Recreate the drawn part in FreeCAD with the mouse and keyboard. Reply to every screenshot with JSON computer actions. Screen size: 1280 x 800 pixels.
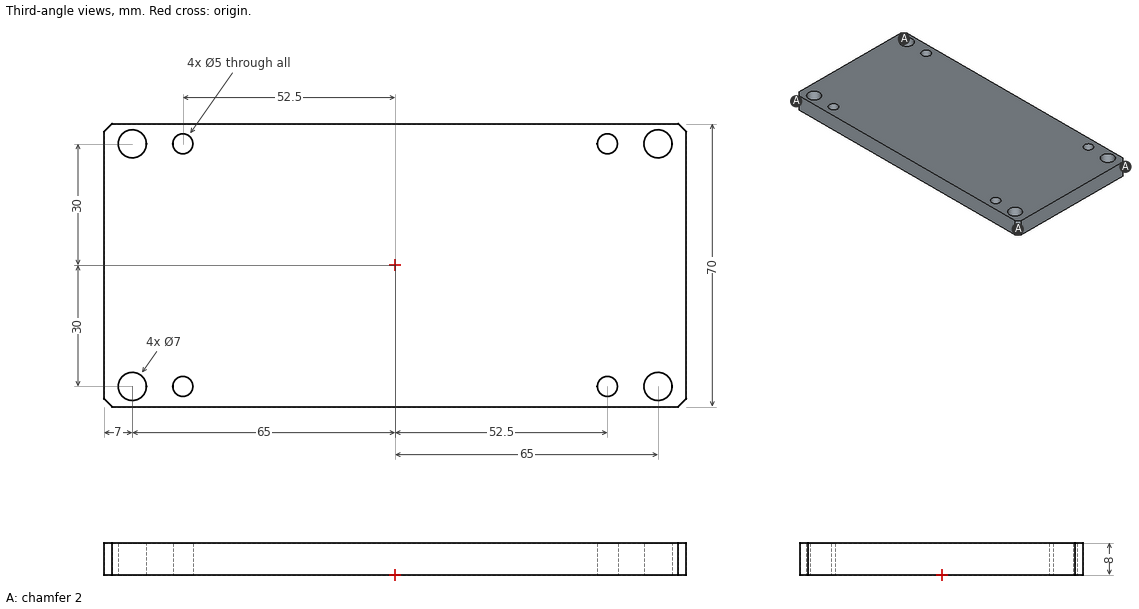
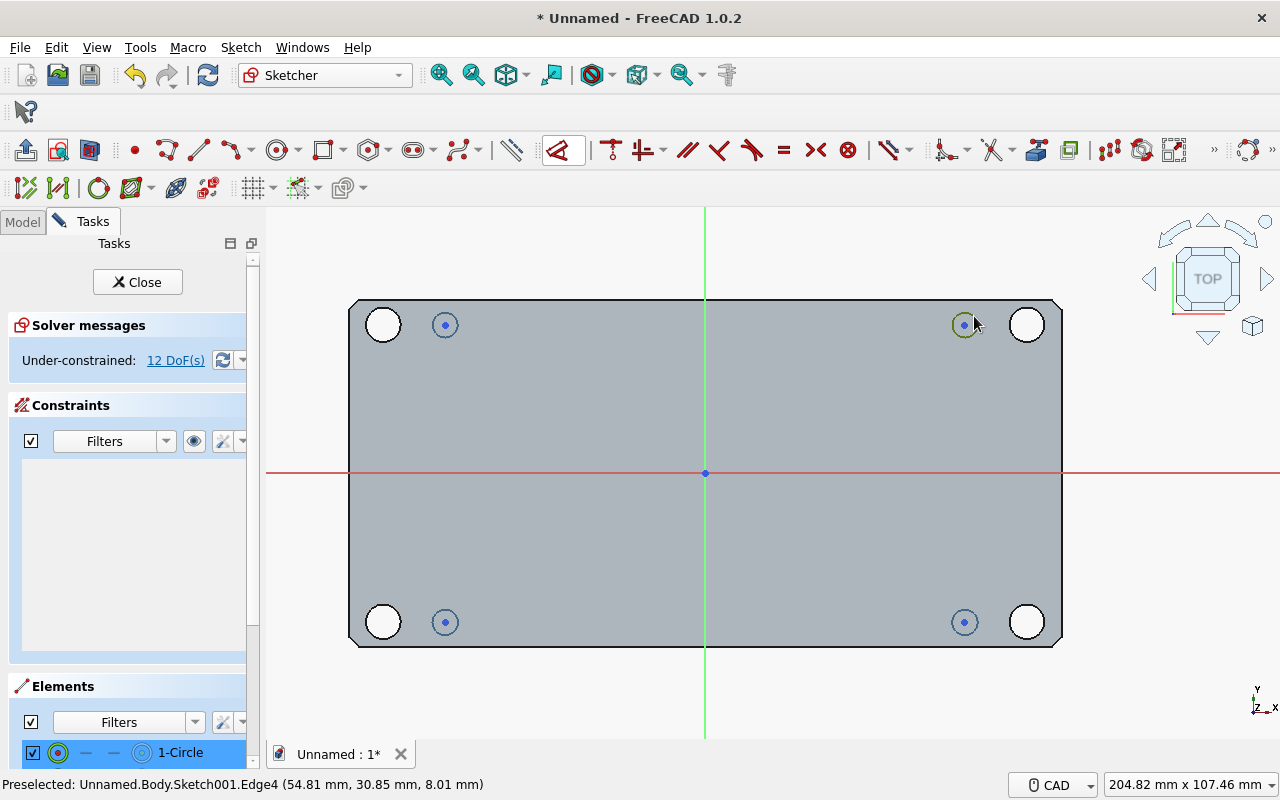
{"action": "left_click", "coordinate": [784, 150]}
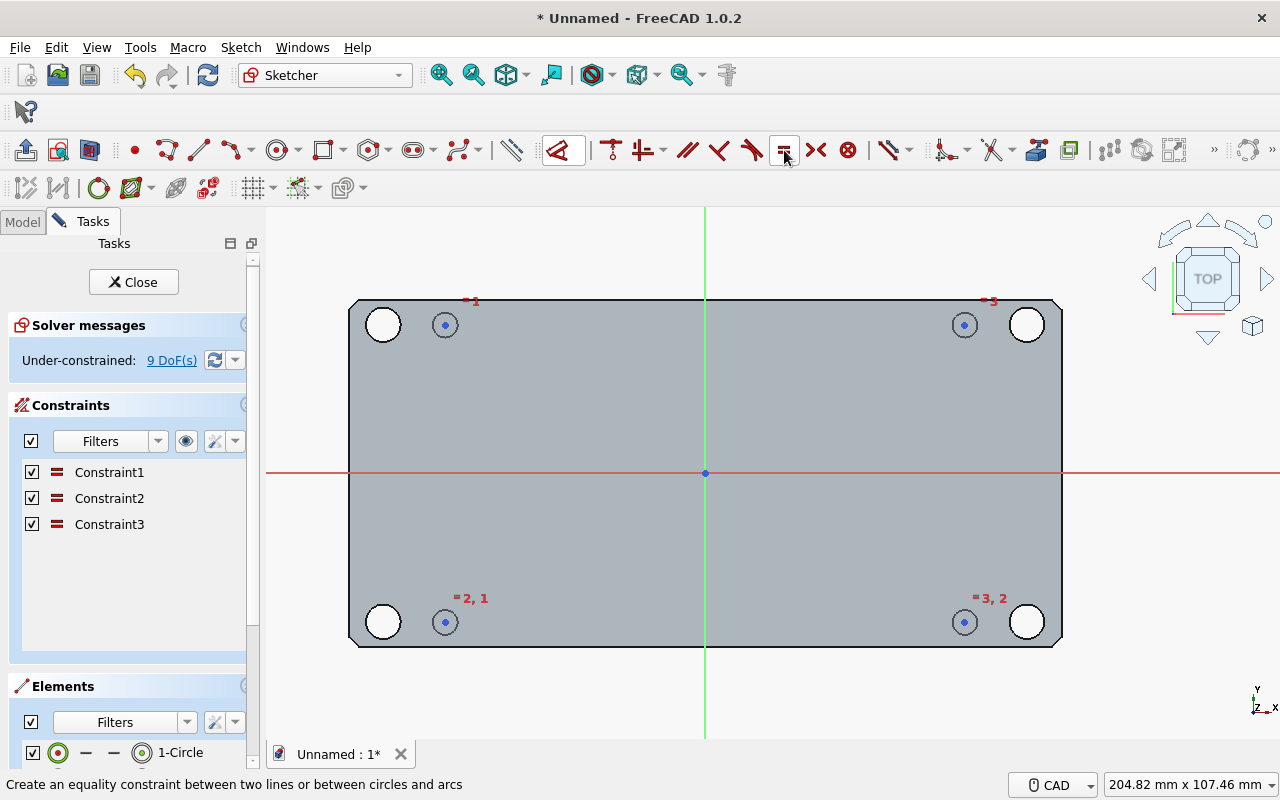
{"action": "scroll", "coordinate": [454, 316], "scroll_direction": "up", "scroll_amount": 3}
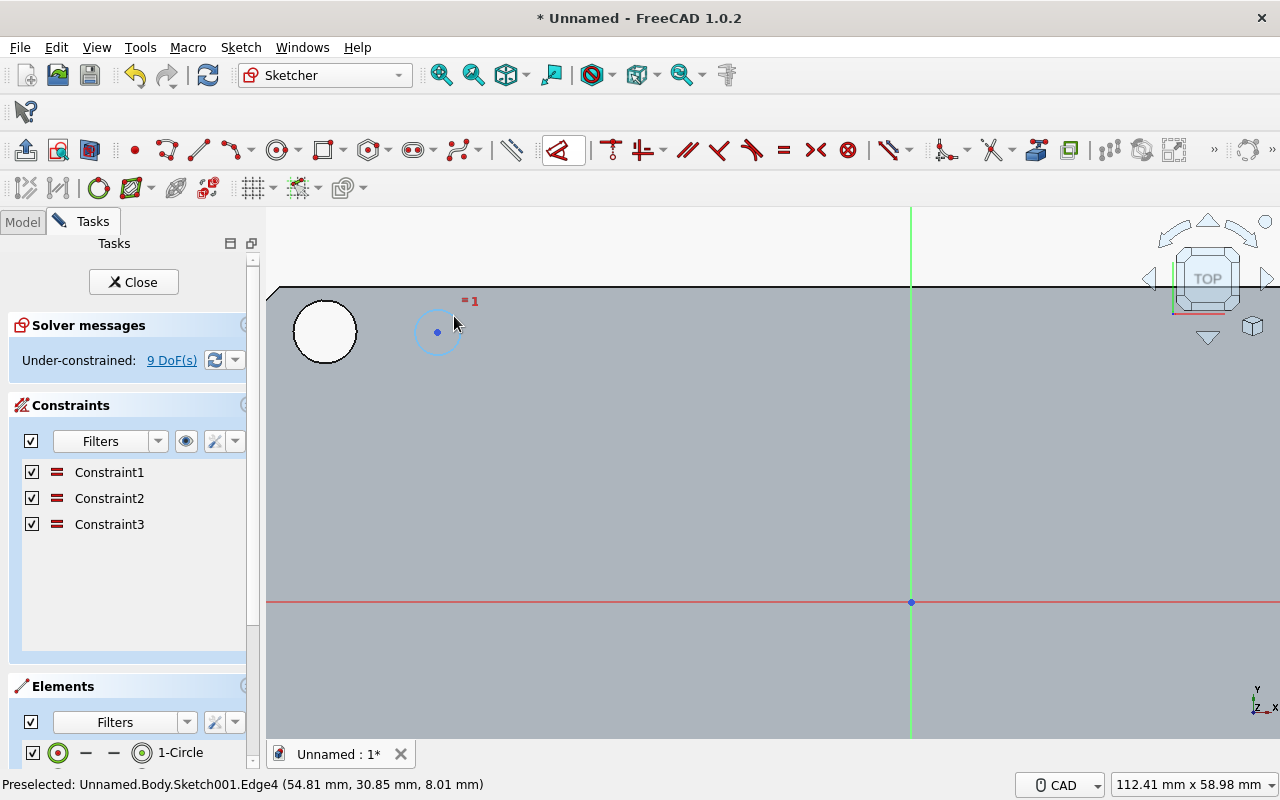
{"action": "left_click", "coordinate": [454, 316]}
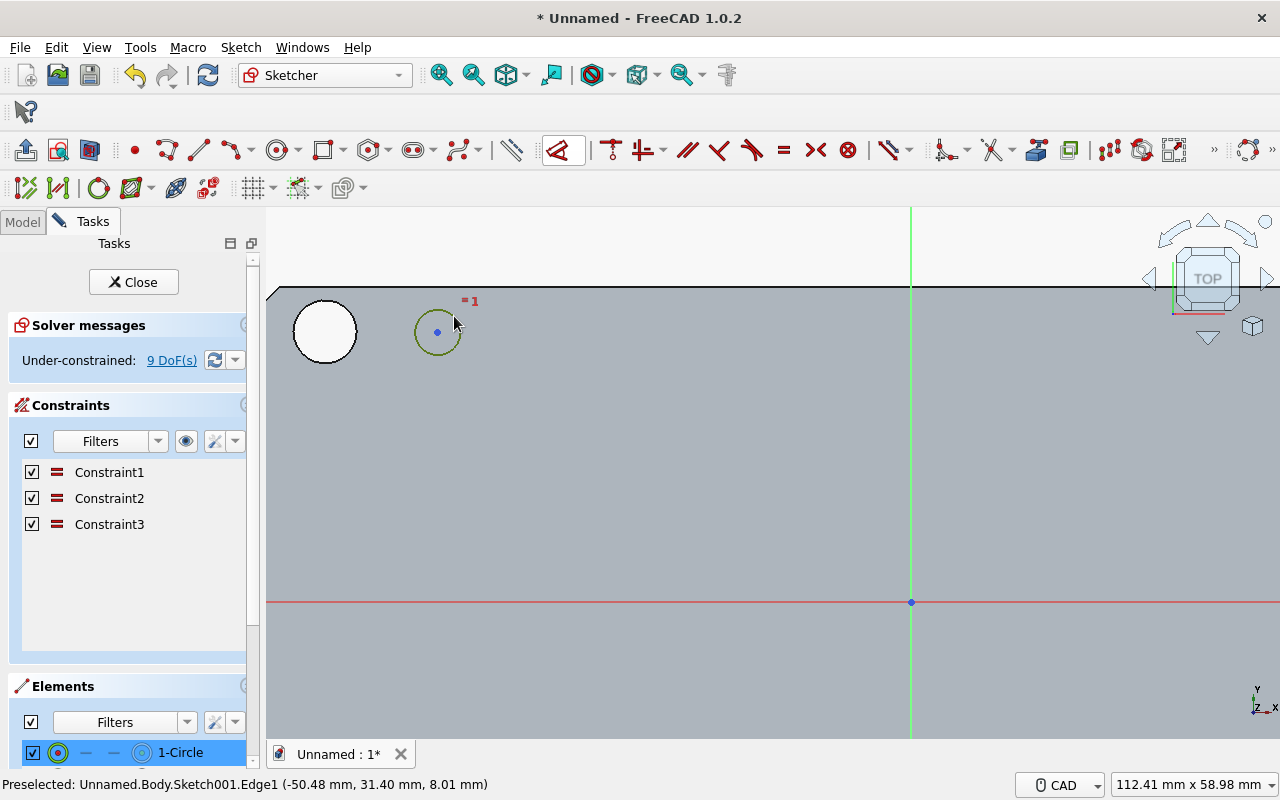
{"action": "key", "text": "k o"}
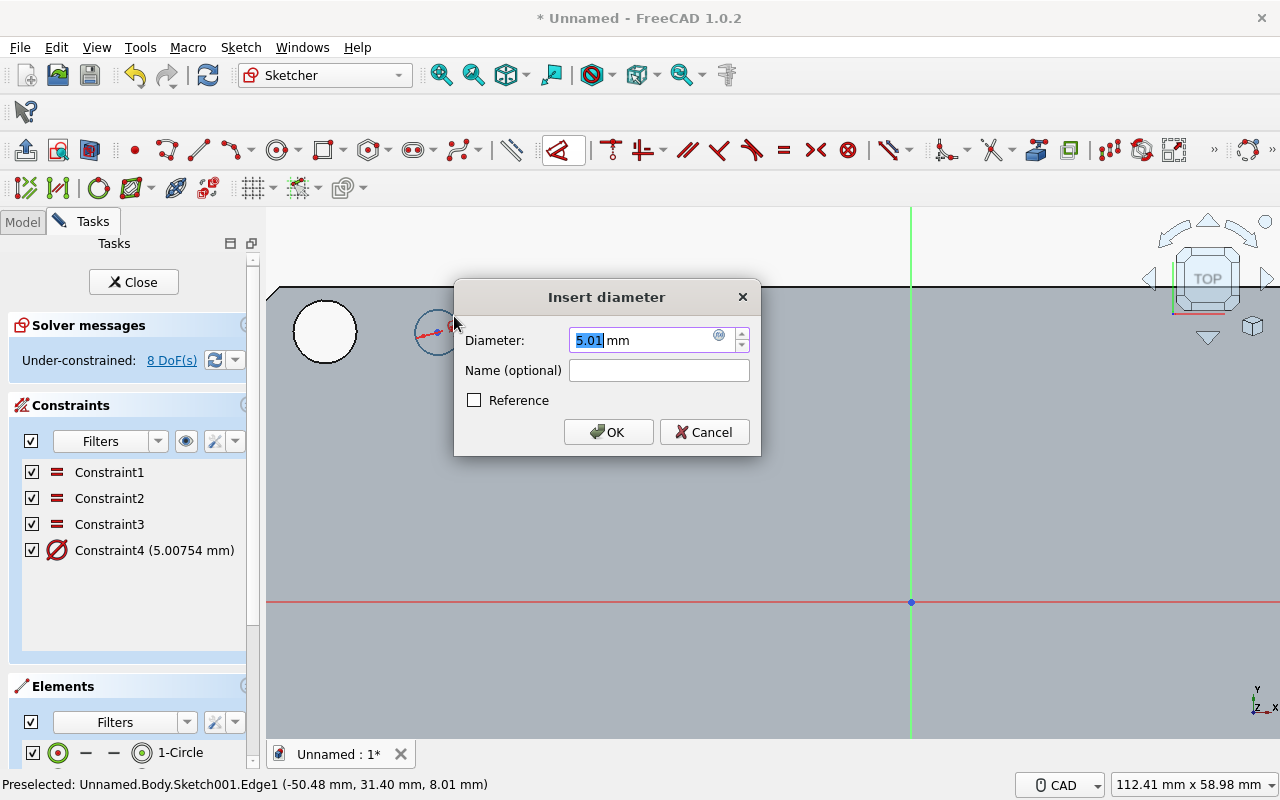
{"action": "type", "text": "5"}
{"action": "key", "text": "Return"}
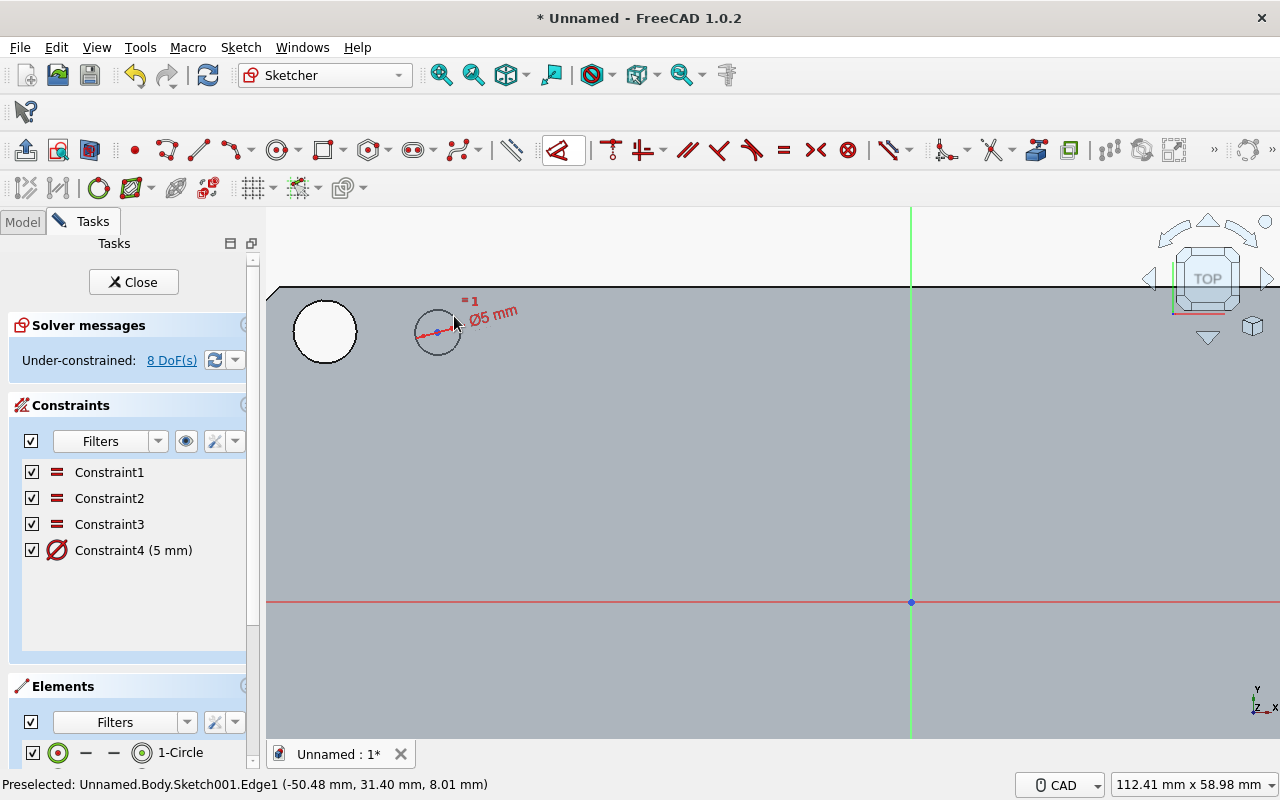
{"action": "left_click", "coordinate": [438, 332]}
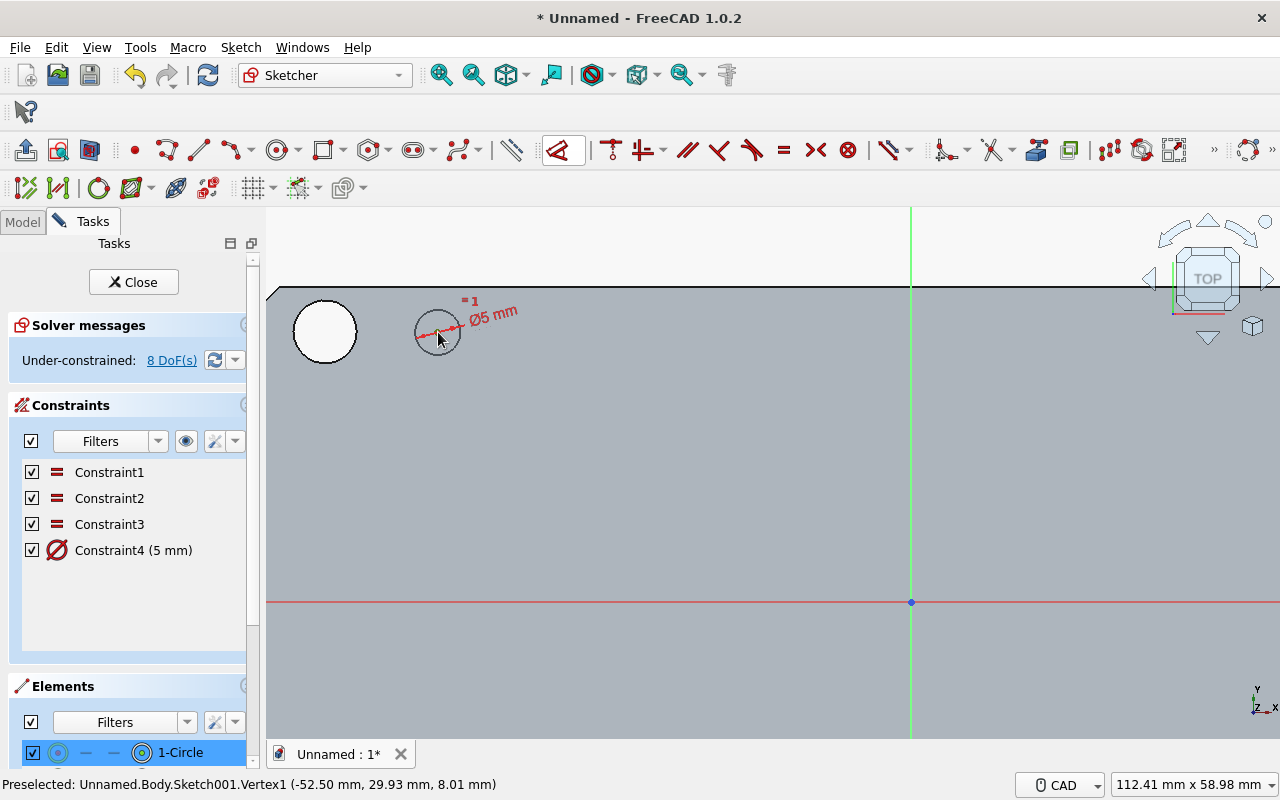
{"action": "left_click", "coordinate": [580, 150]}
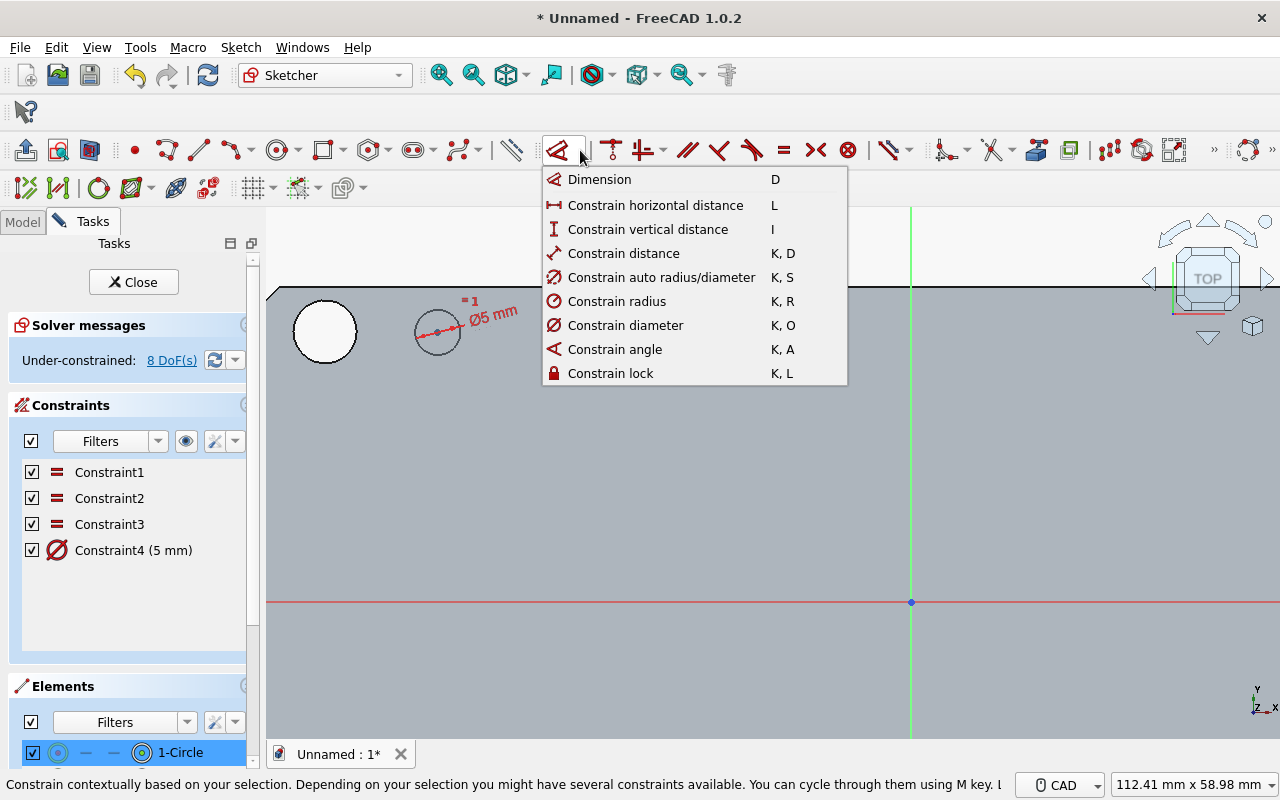
{"action": "left_click", "coordinate": [695, 229]}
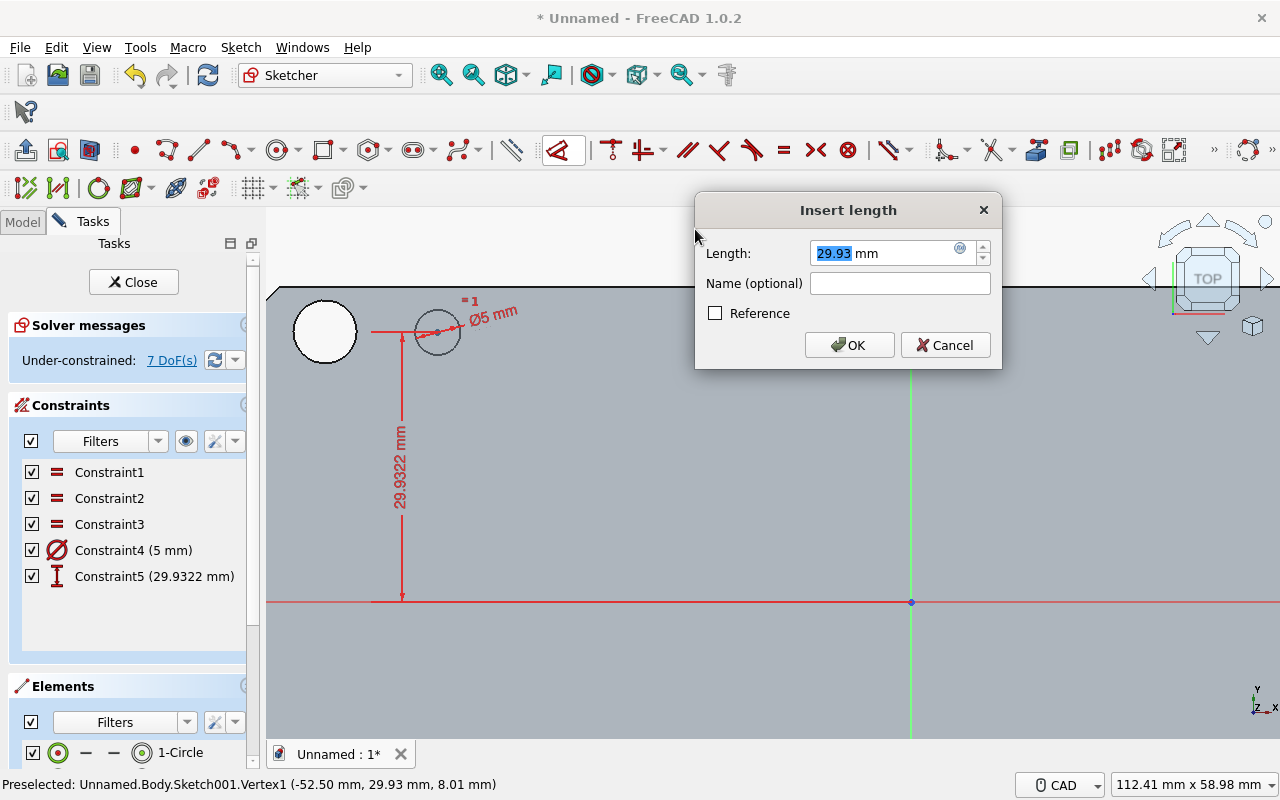
{"action": "type", "text": "30"}
{"action": "key", "text": "Return"}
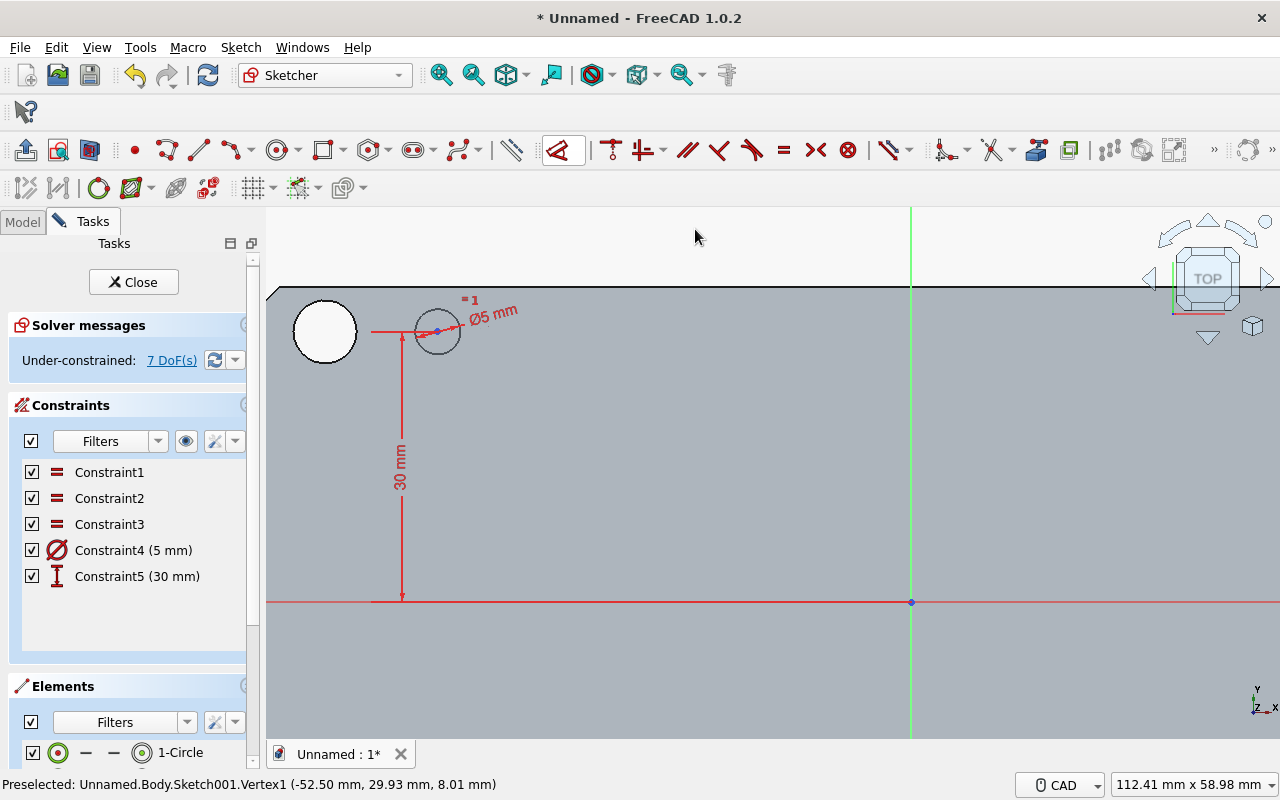
{"action": "scroll", "coordinate": [453, 316], "scroll_direction": "down", "scroll_amount": 3}